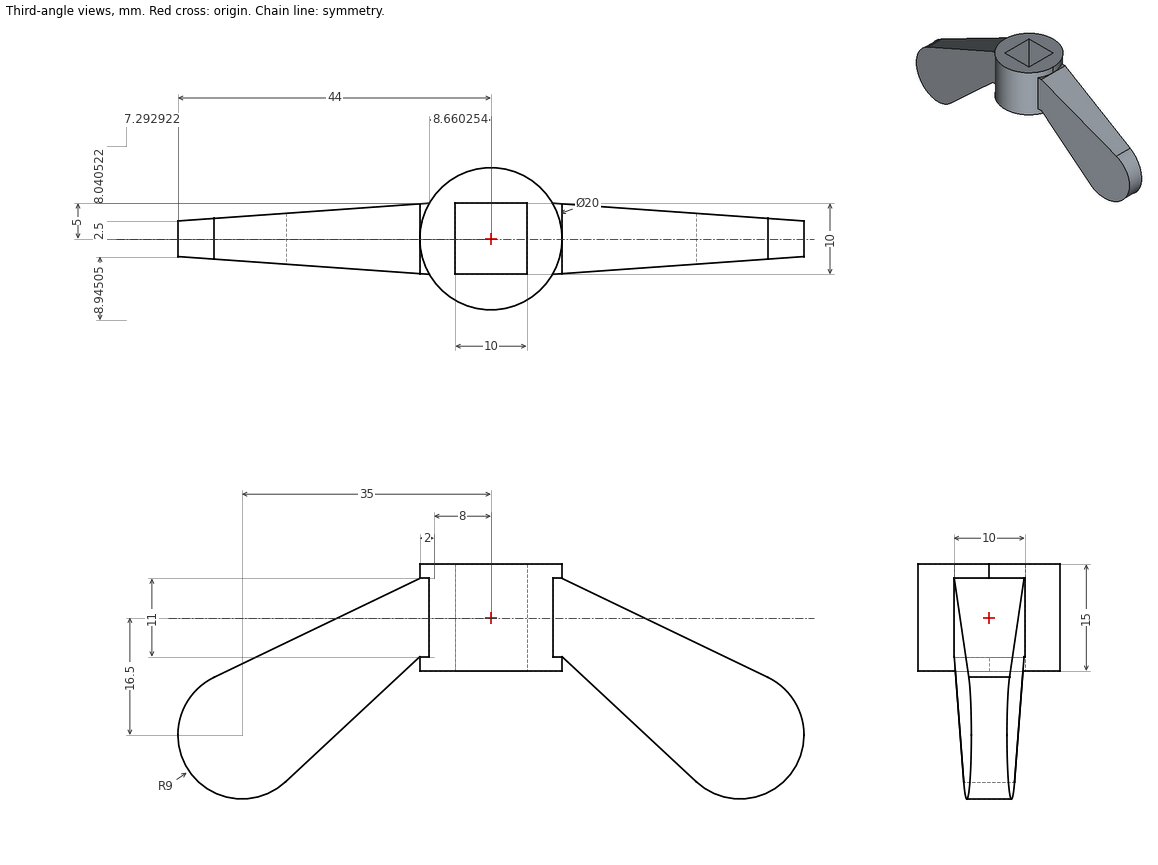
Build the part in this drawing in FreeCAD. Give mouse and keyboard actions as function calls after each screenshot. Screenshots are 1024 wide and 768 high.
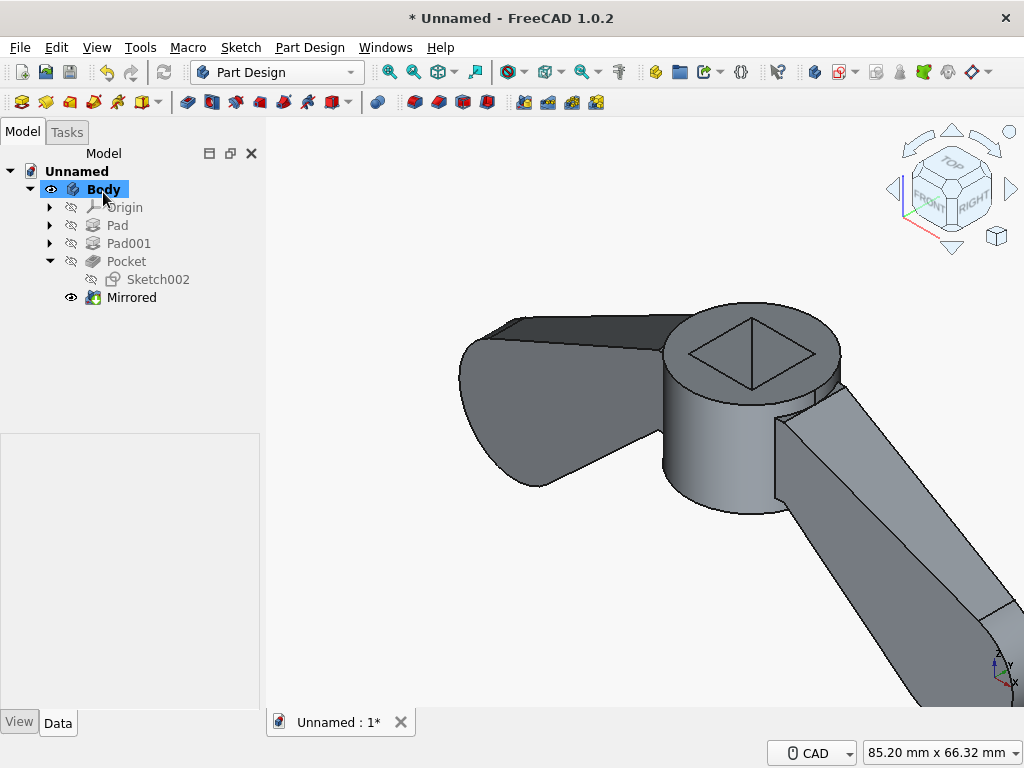
key(v)
key(f)